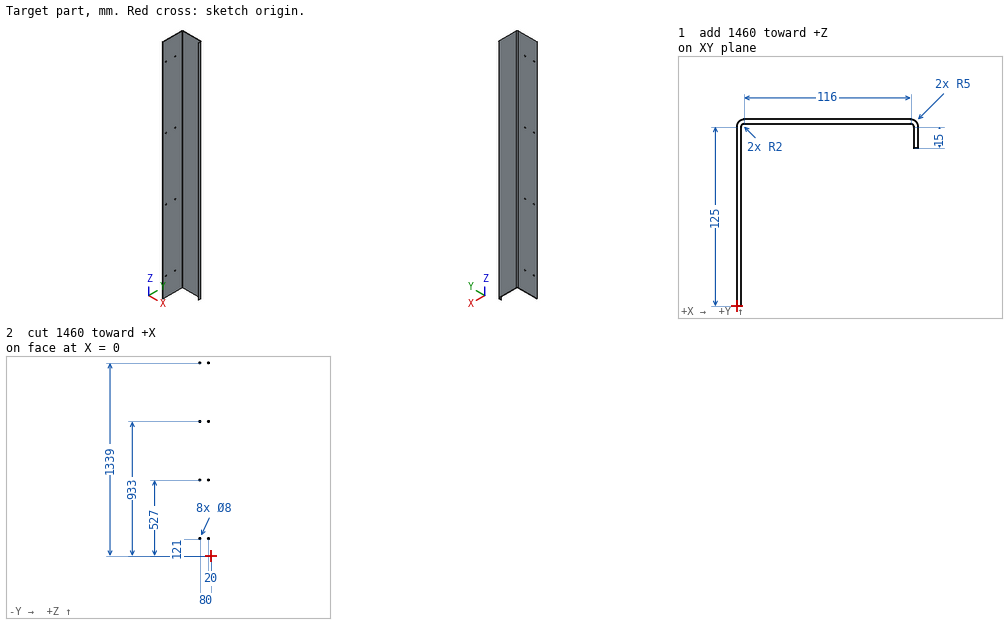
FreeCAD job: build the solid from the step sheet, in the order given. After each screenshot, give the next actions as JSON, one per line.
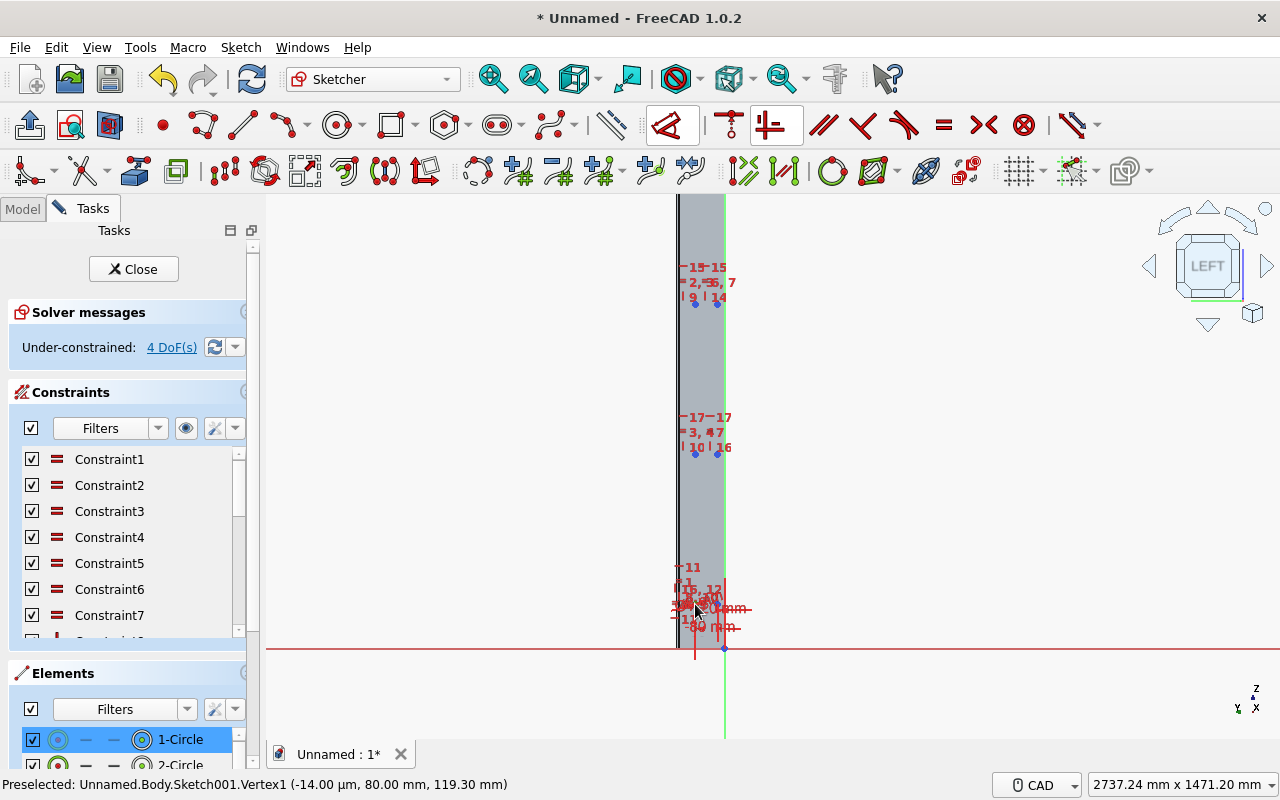
{"action": "key", "text": "i"}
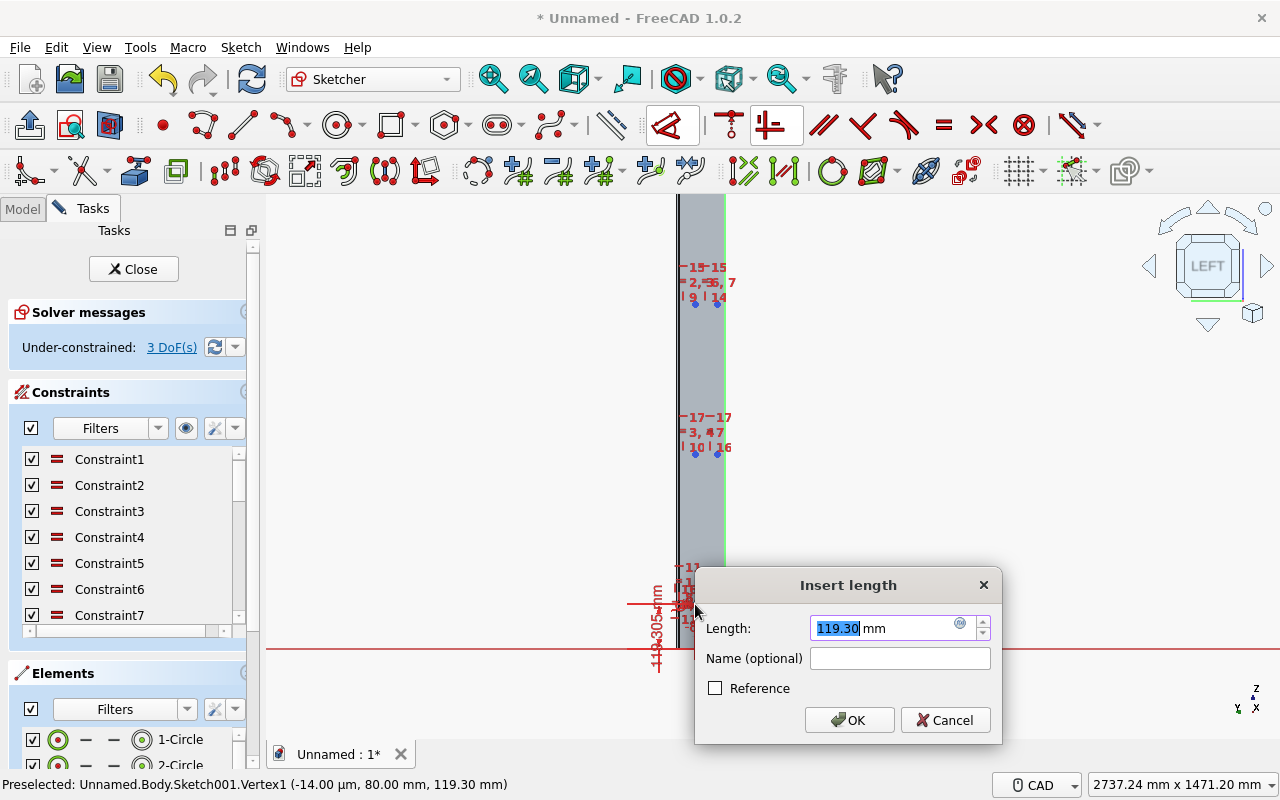
{"action": "type", "text": "121"}
{"action": "key", "text": "Return"}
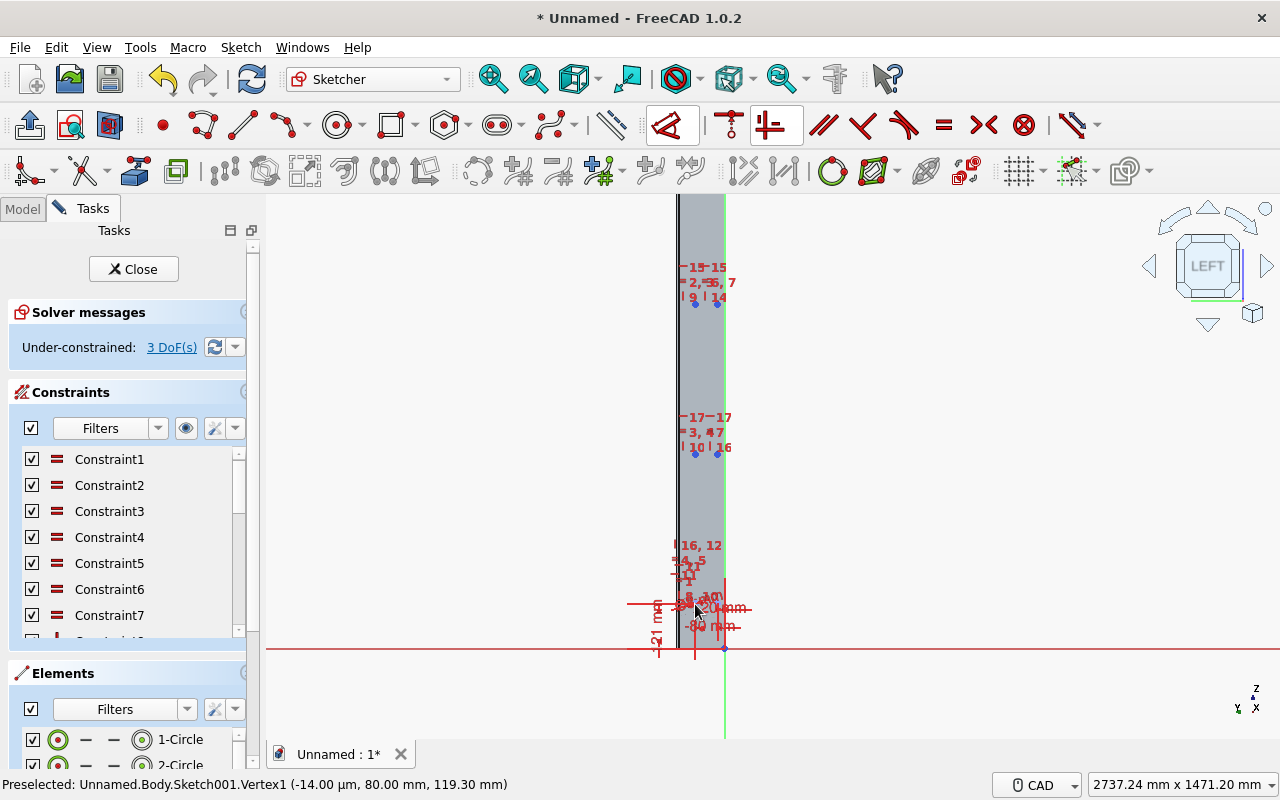
{"action": "left_click", "coordinate": [695, 304]}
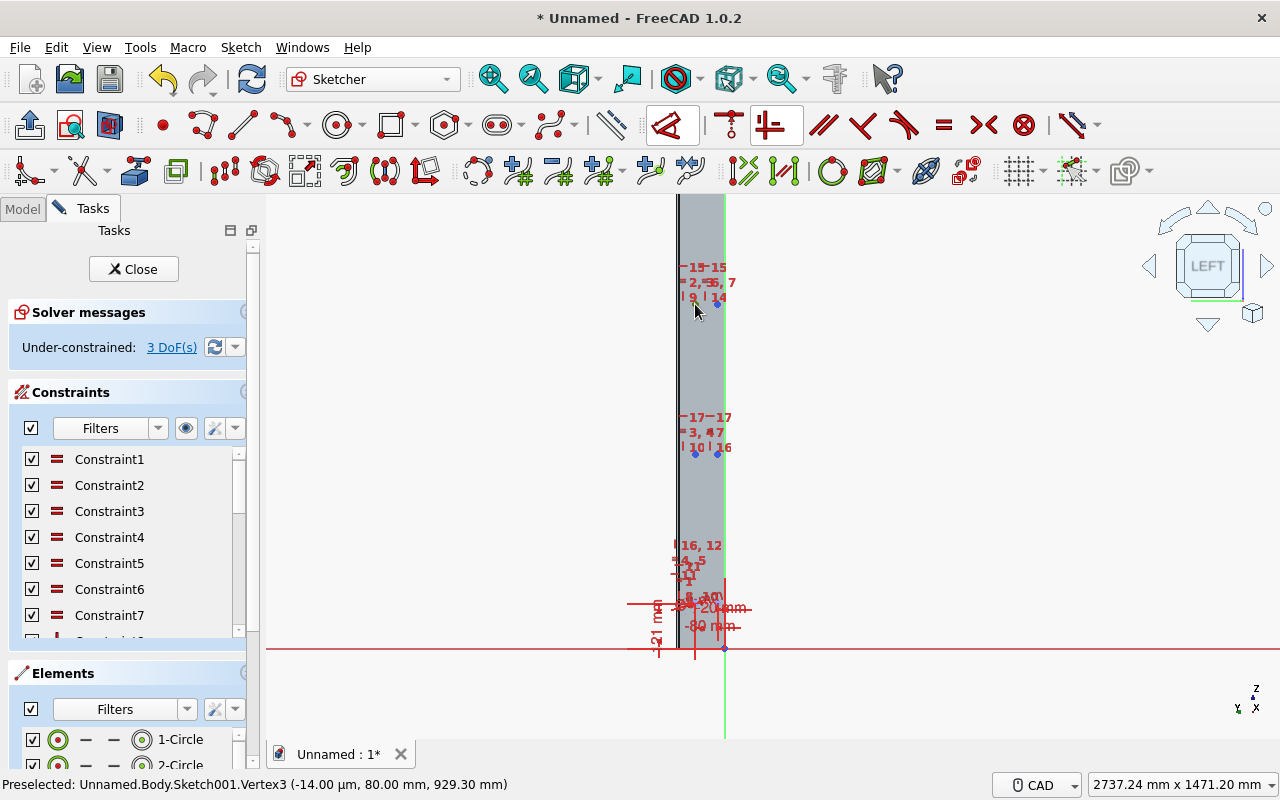
{"action": "key", "text": "i"}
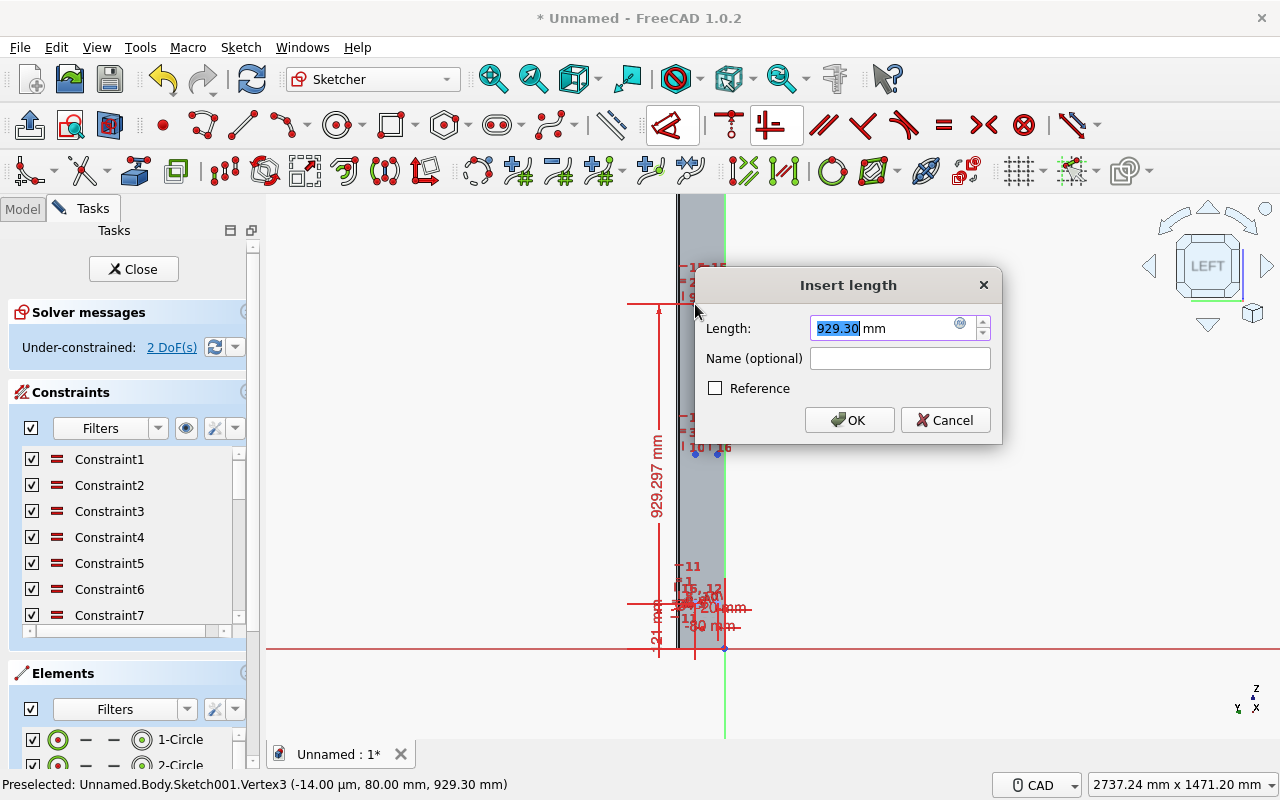
{"action": "type", "text": "933"}
{"action": "key", "text": "Return"}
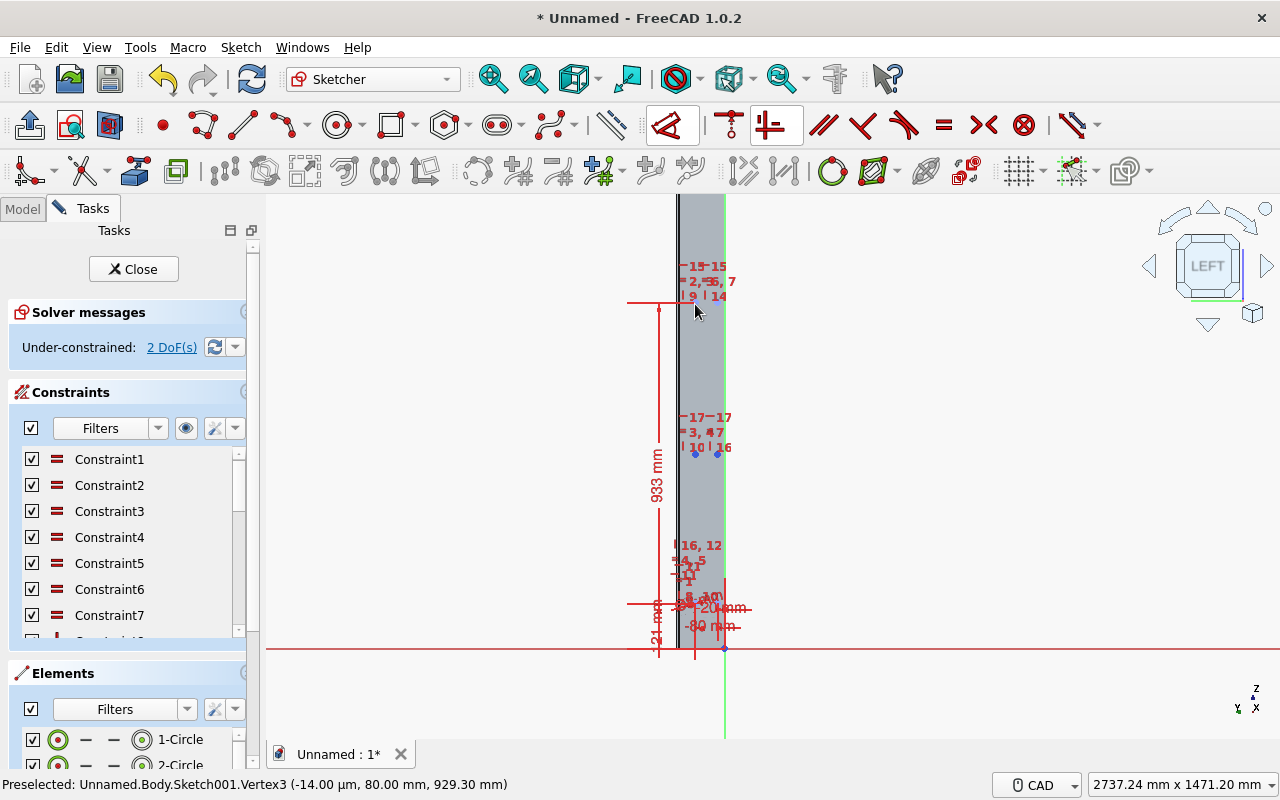
{"action": "left_click", "coordinate": [695, 454]}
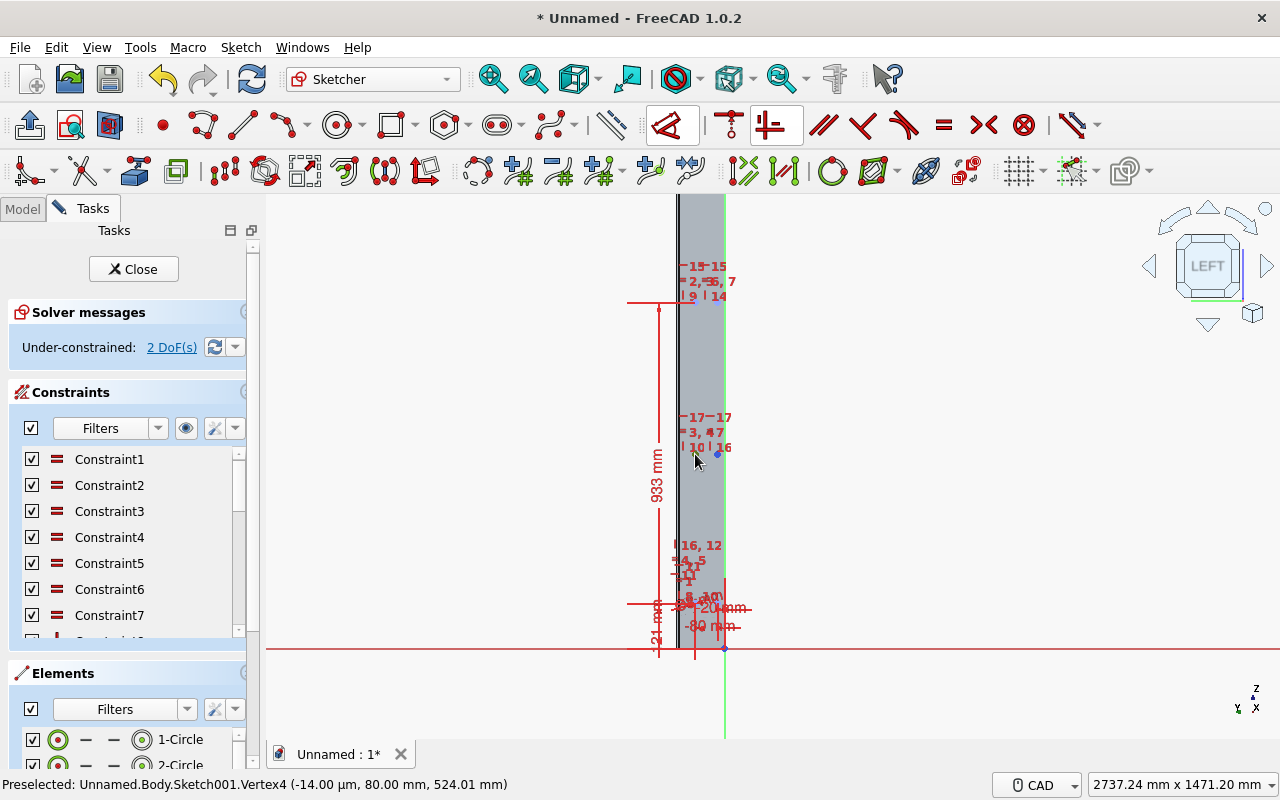
{"action": "key", "text": "i"}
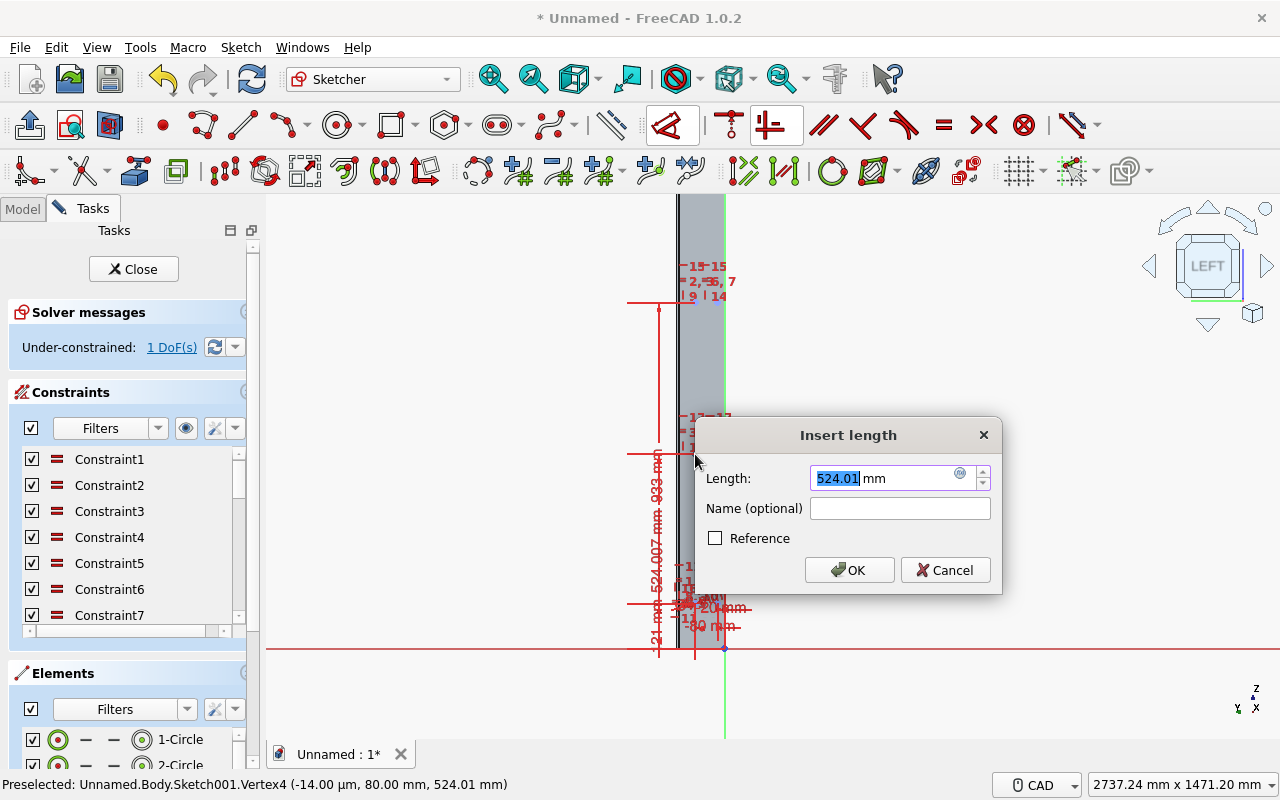
{"action": "type", "text": "527"}
{"action": "key", "text": "Return"}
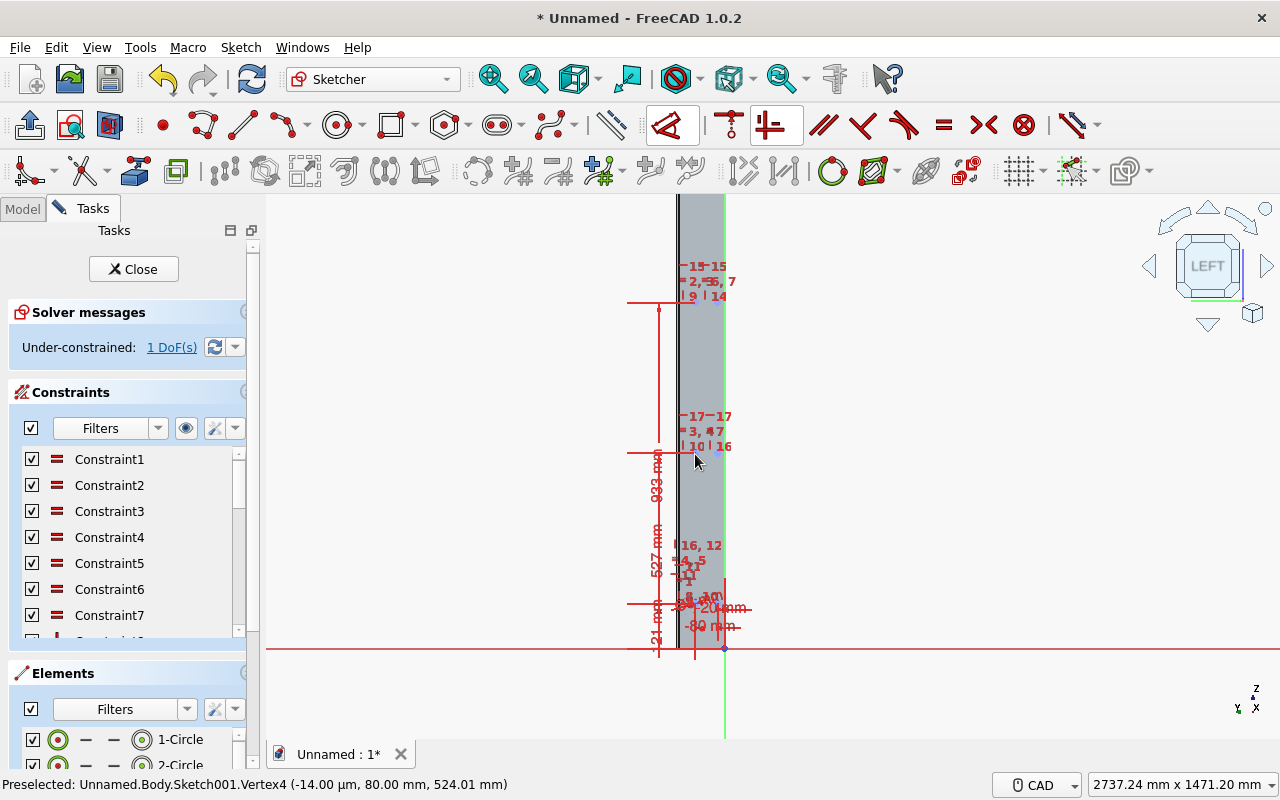
{"action": "scroll", "coordinate": [694, 602], "scroll_direction": "down", "scroll_amount": 2}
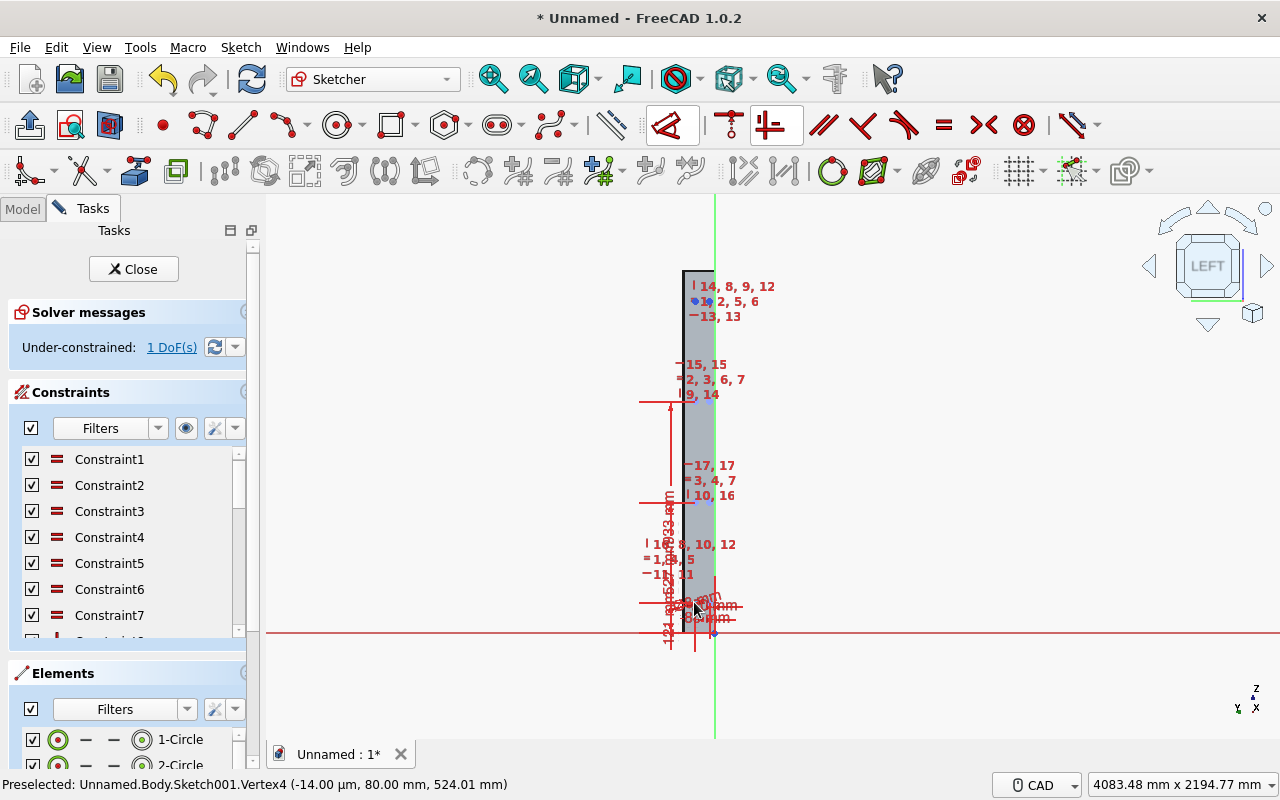
{"action": "left_click", "coordinate": [695, 302]}